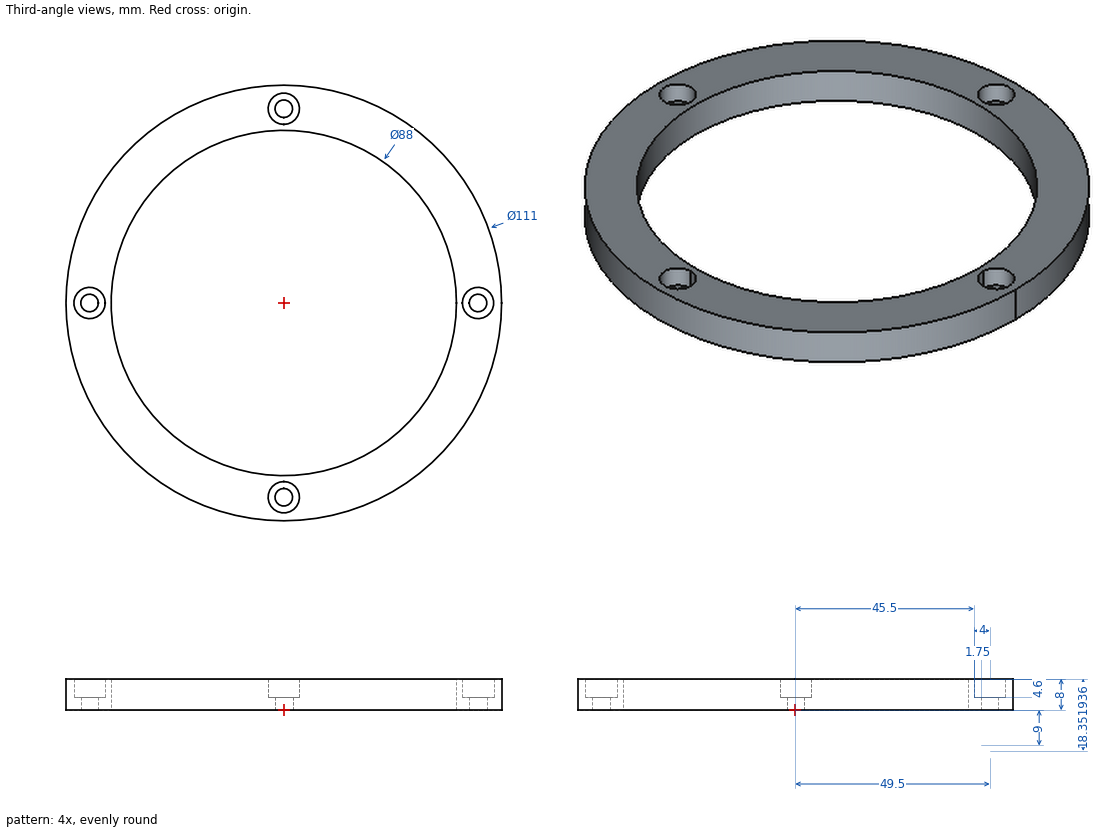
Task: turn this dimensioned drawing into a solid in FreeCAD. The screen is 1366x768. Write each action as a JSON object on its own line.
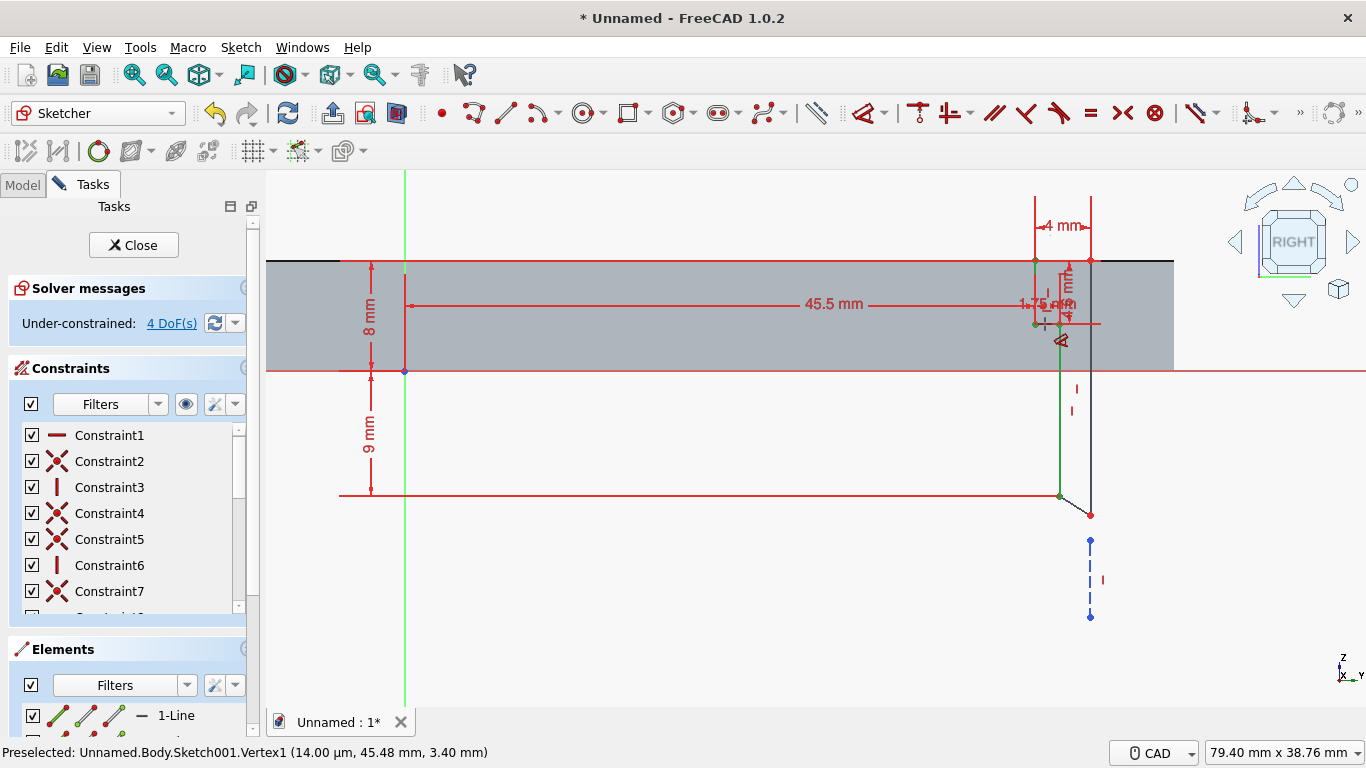
{"action": "left_click", "coordinate": [1090, 541]}
{"action": "left_click", "coordinate": [748, 575]}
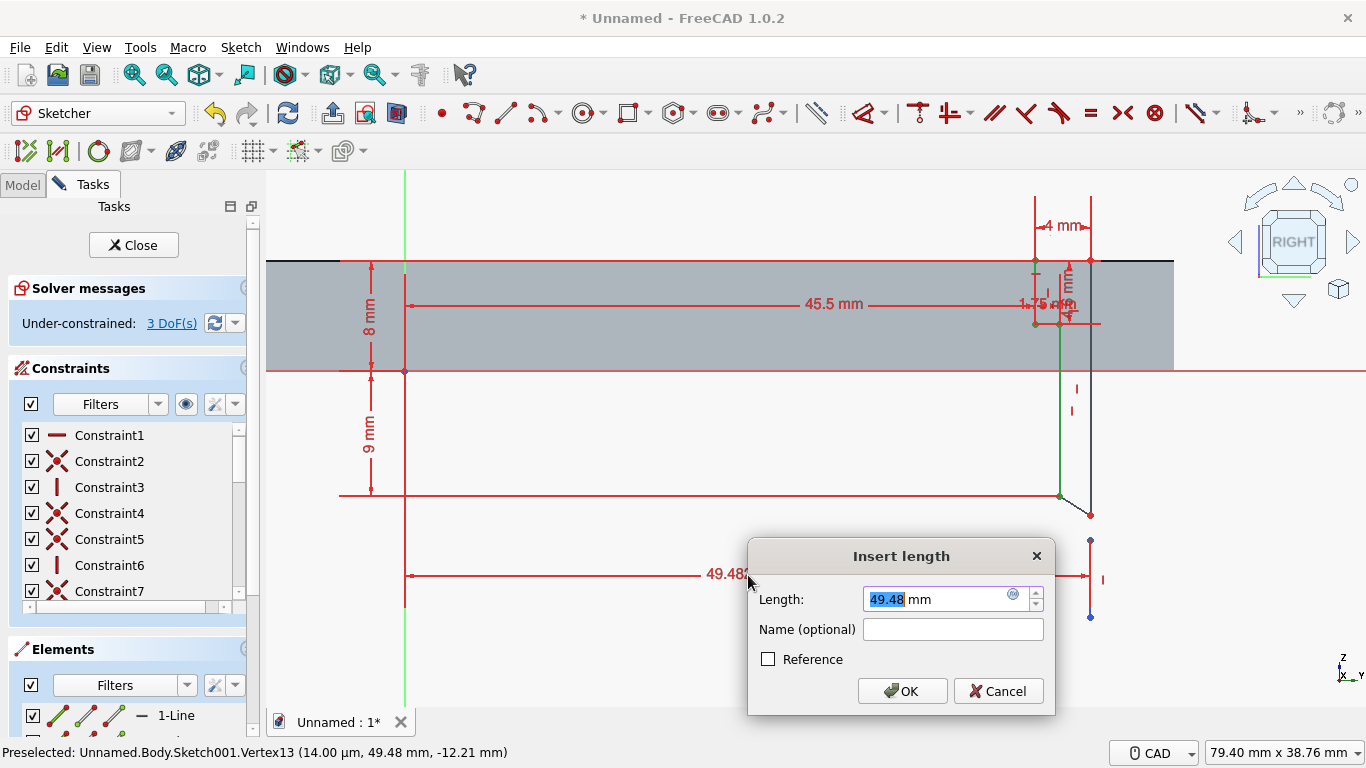
{"action": "type", "text": "49.5"}
{"action": "key", "text": "Return"}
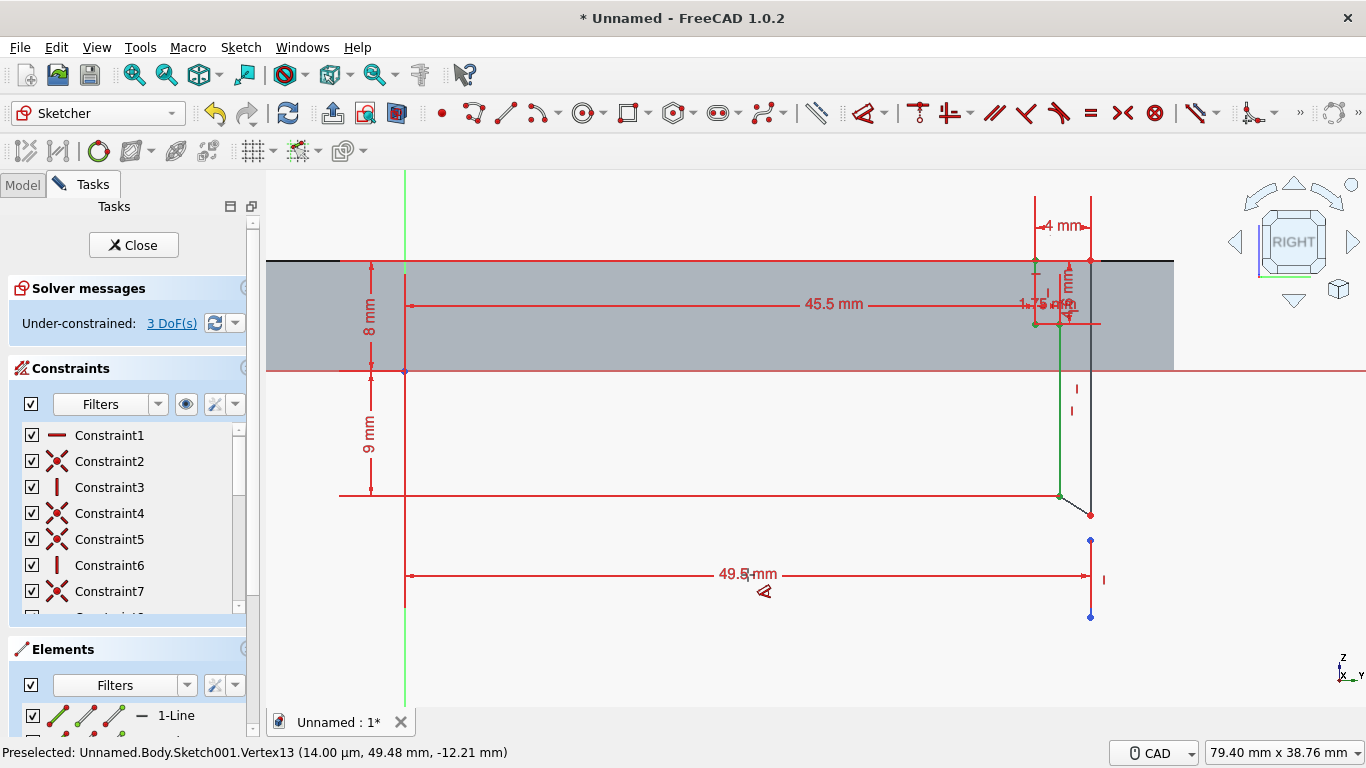
{"action": "left_click", "coordinate": [1091, 439]}
{"action": "left_click", "coordinate": [1125, 388]}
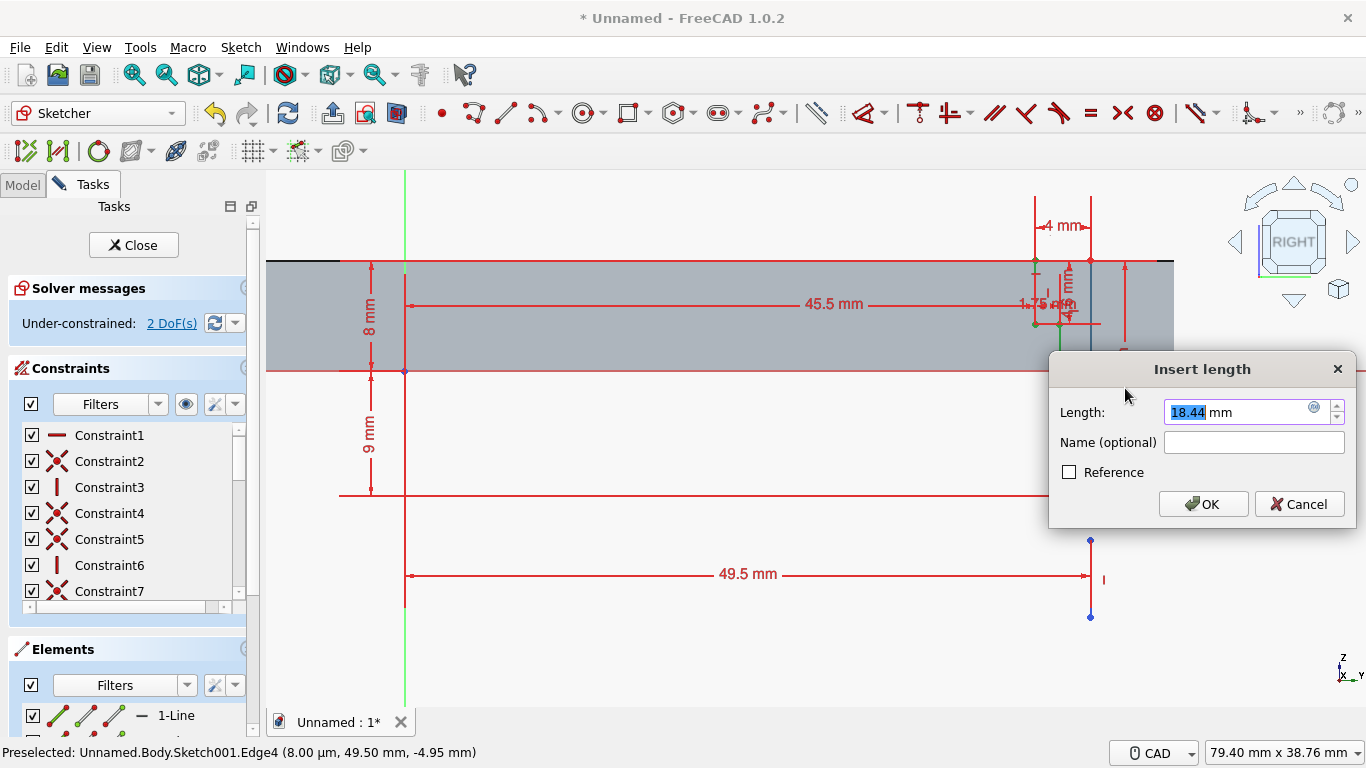
{"action": "type", "text": "18.351936"}
{"action": "key", "text": "Return"}
{"action": "key", "text": "Escape"}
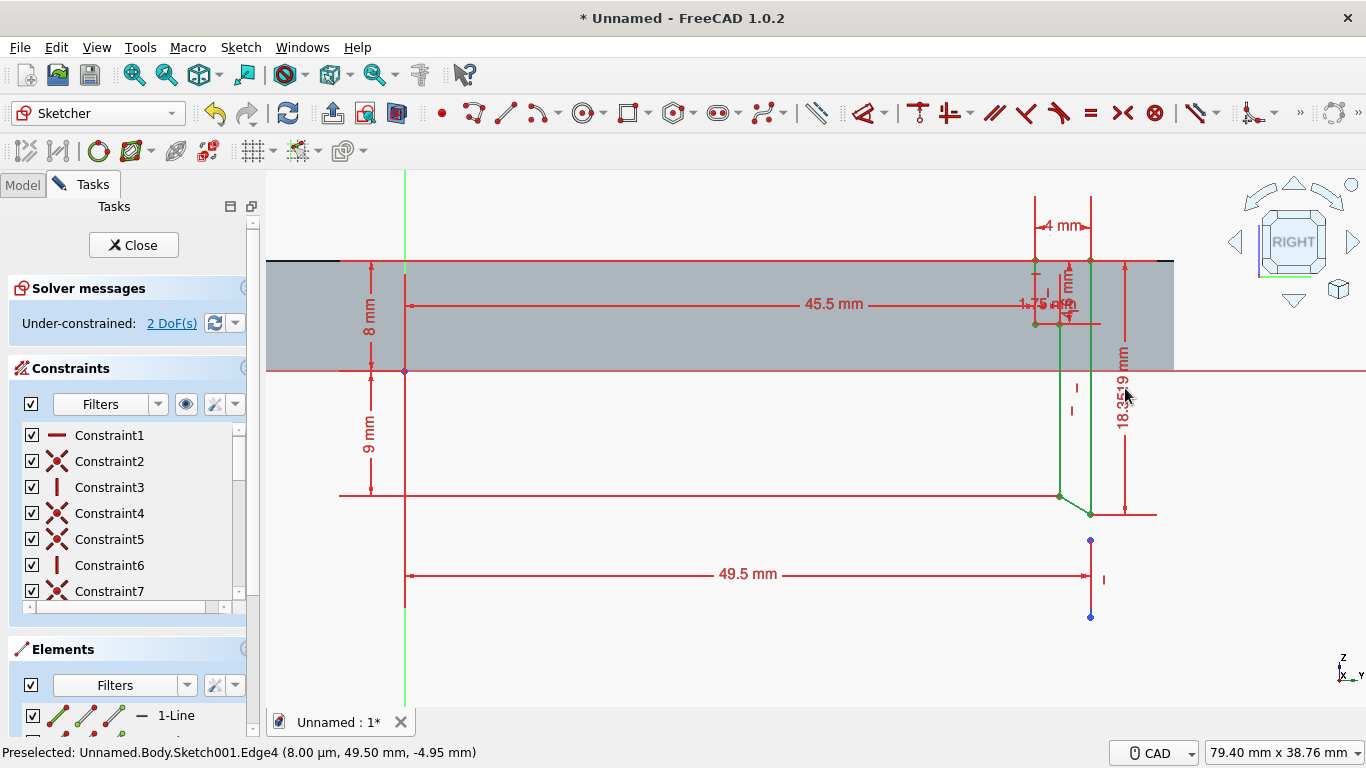
{"action": "left_click", "coordinate": [134, 245]}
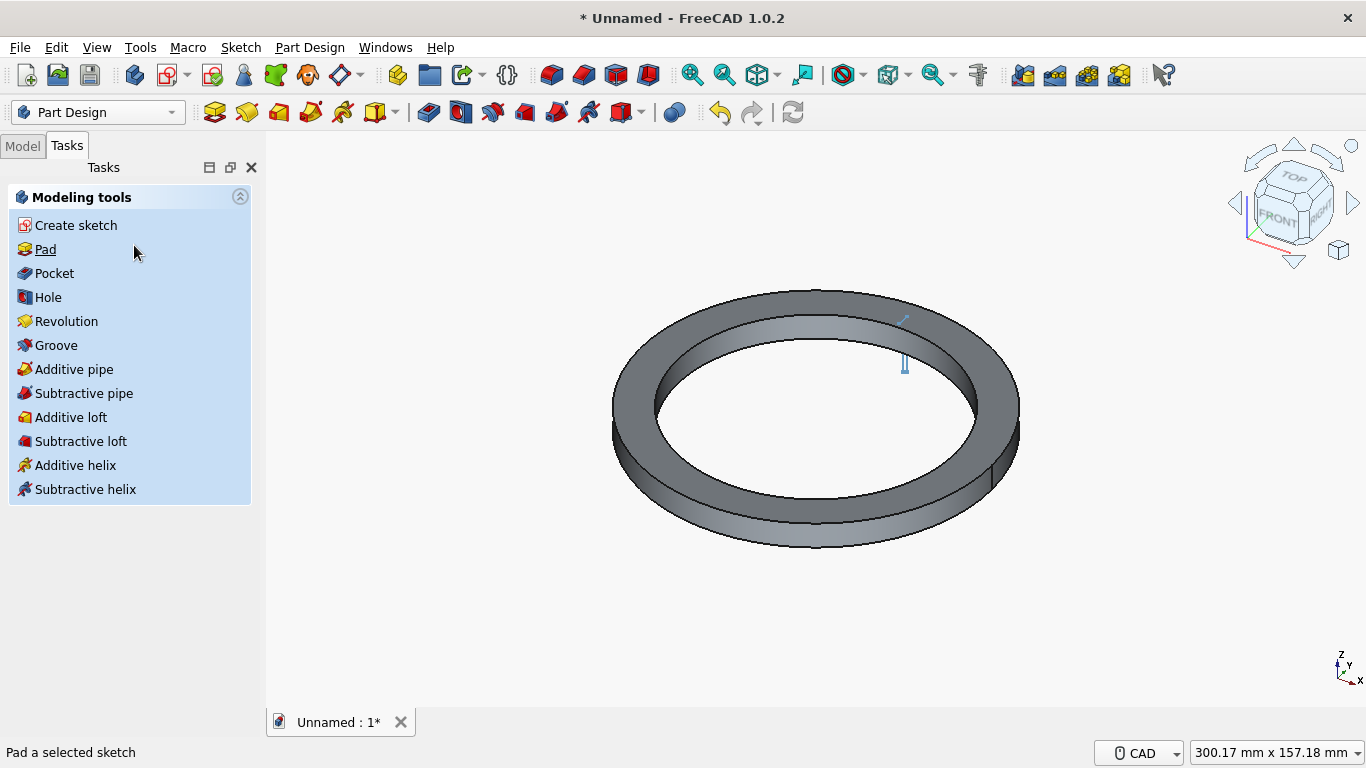
{"action": "left_click", "coordinate": [494, 112]}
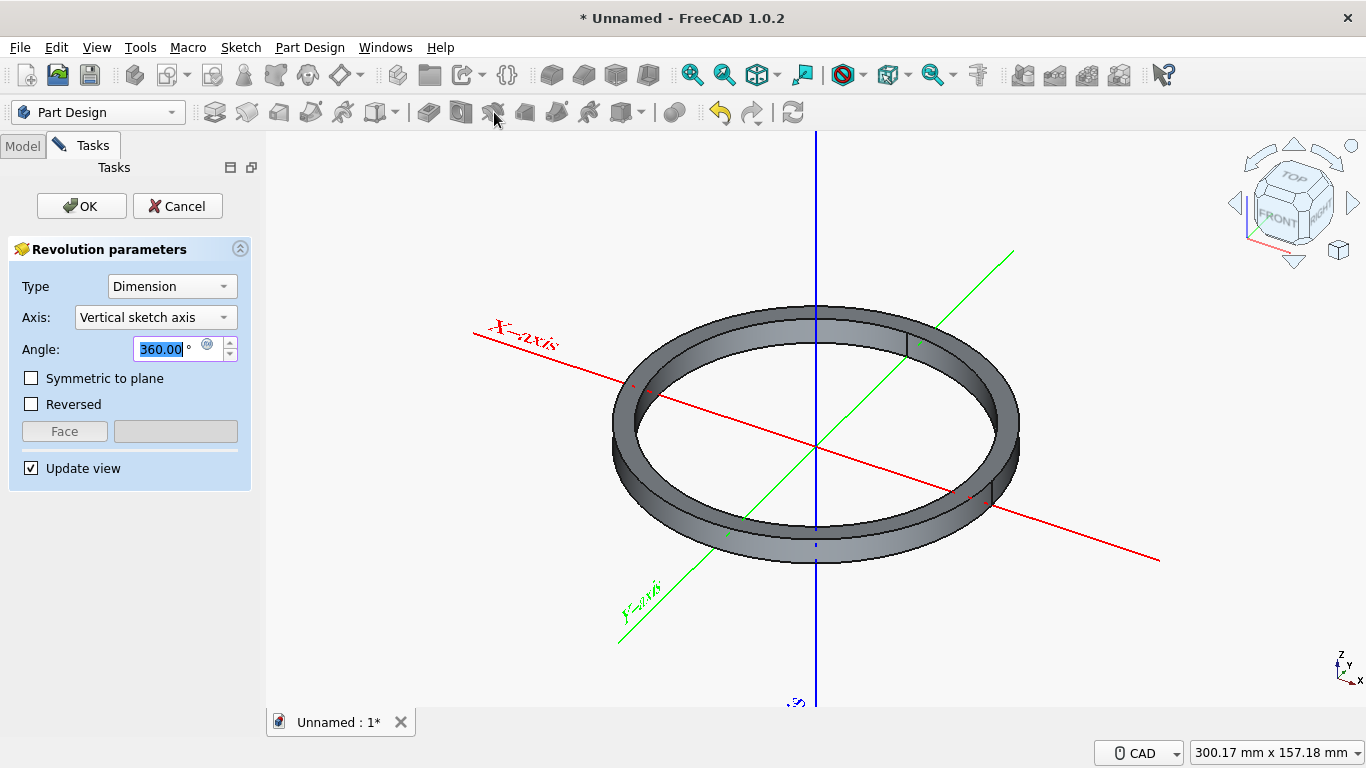
{"action": "left_click", "coordinate": [156, 318]}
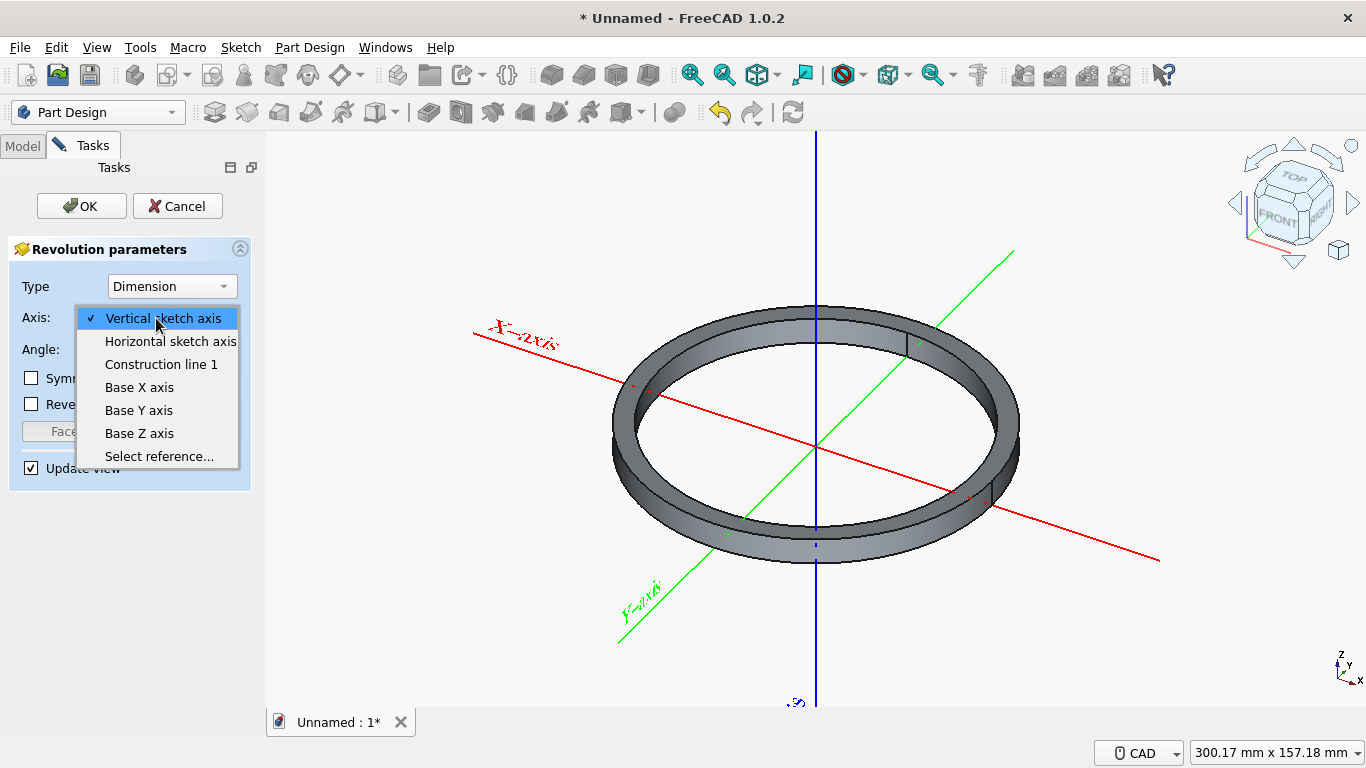
{"action": "left_click", "coordinate": [156, 364]}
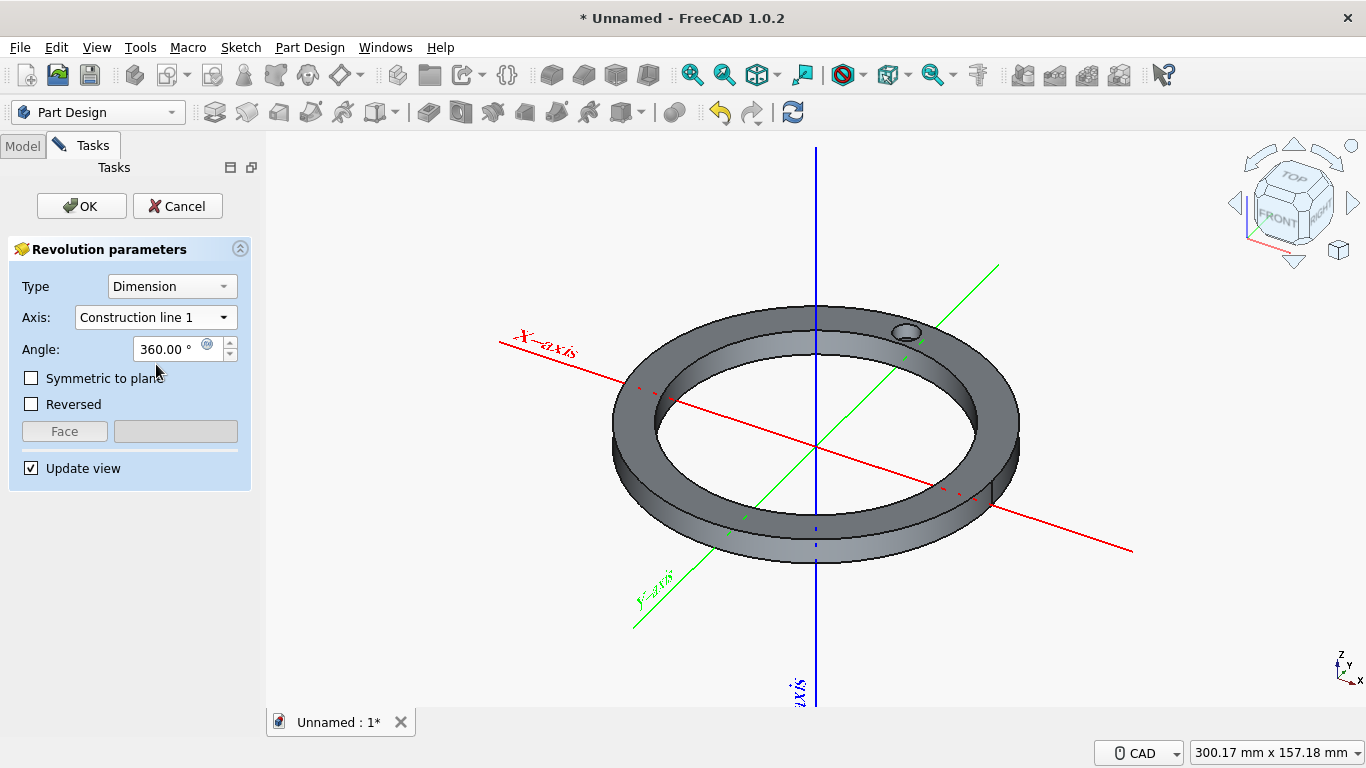
{"action": "left_click", "coordinate": [82, 206]}